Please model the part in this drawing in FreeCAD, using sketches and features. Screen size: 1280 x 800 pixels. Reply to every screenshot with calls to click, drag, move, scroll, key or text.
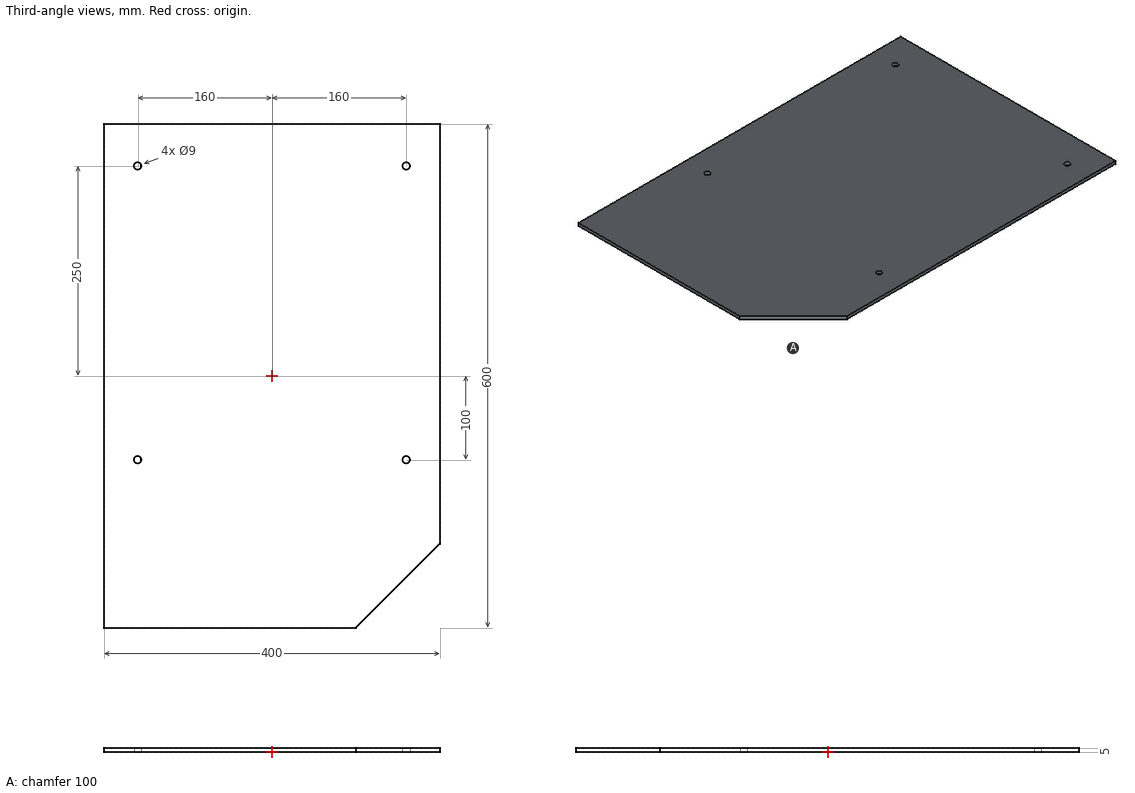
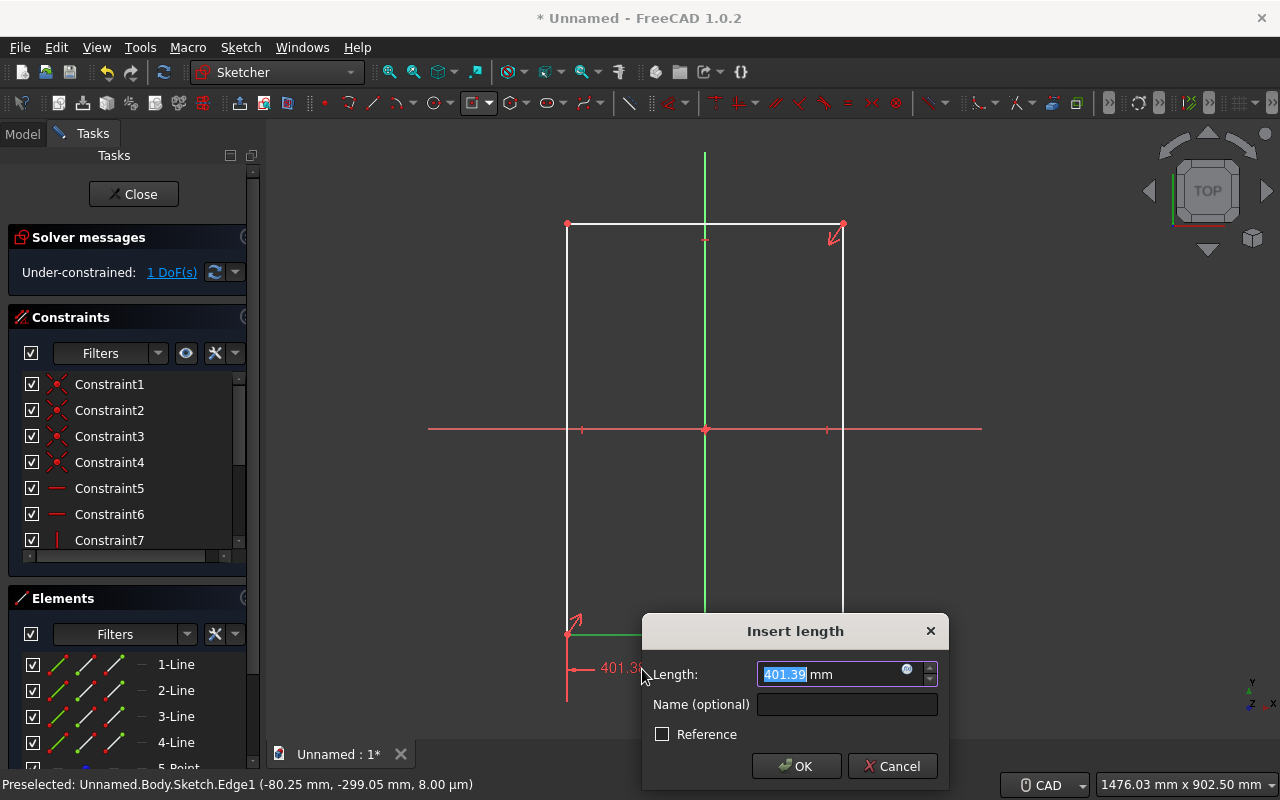
text(400)
key(Return)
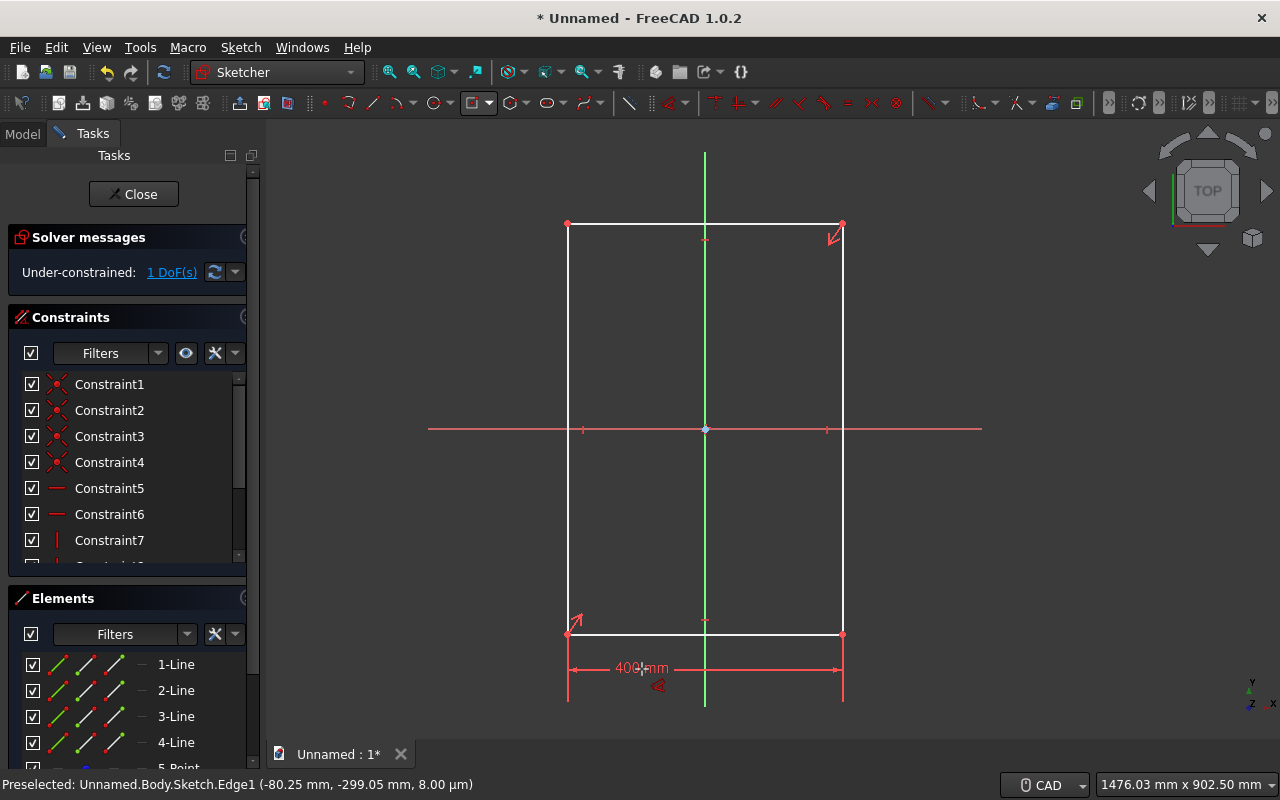
click(843, 512)
click(877, 335)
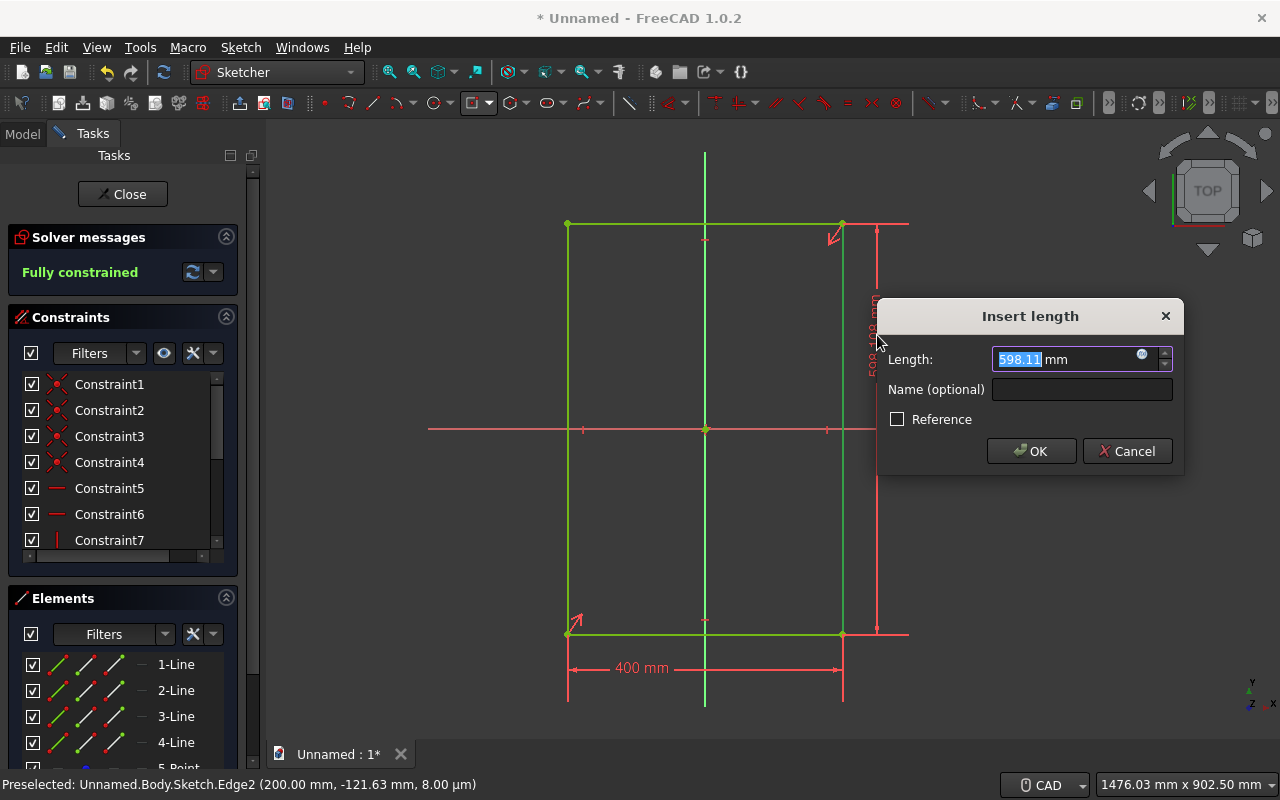
text(600)
key(Return)
key(Escape)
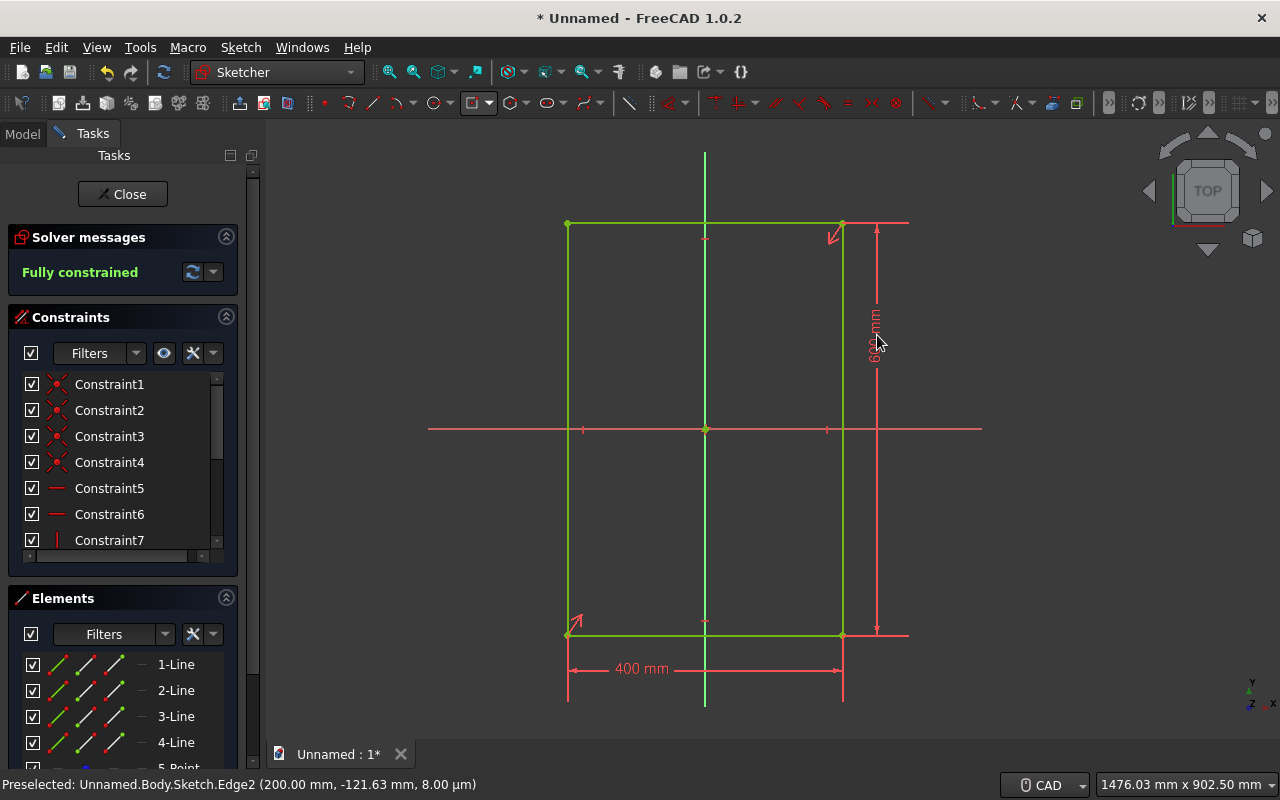
click(123, 194)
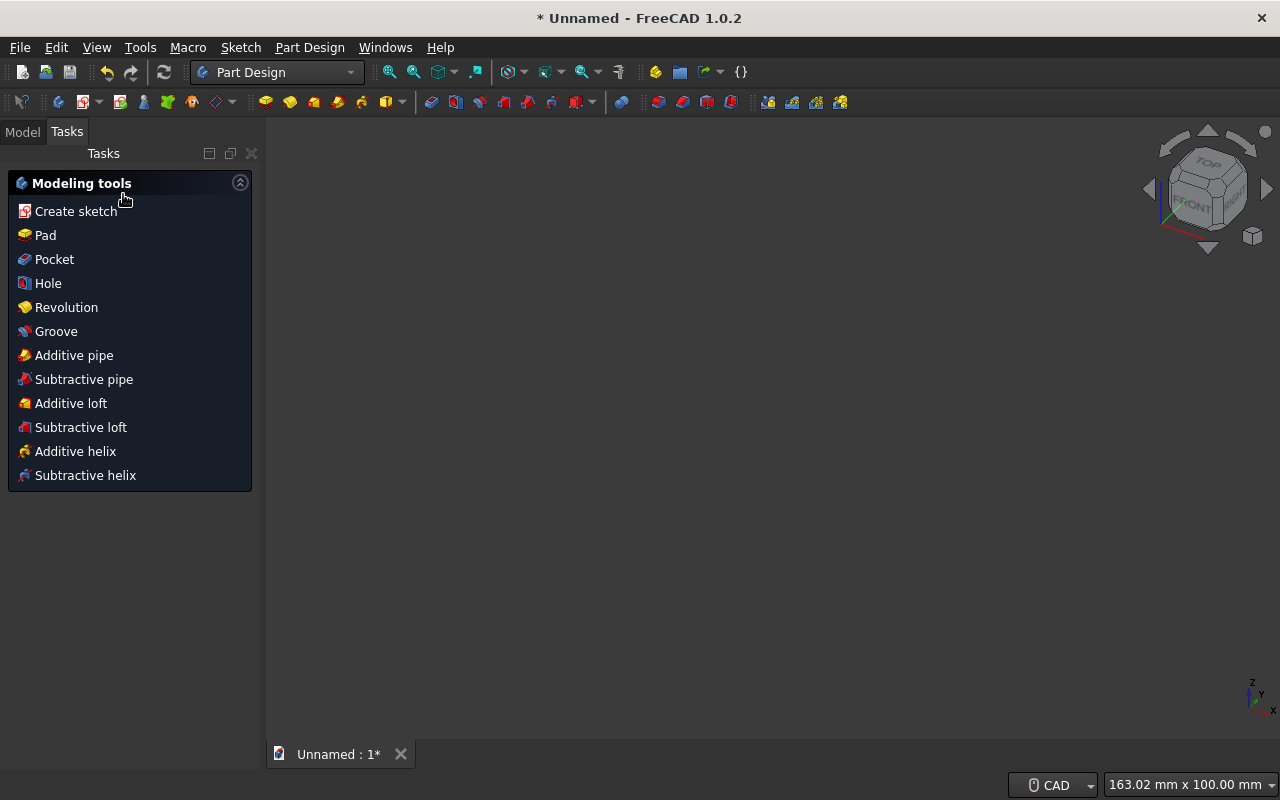
click(266, 102)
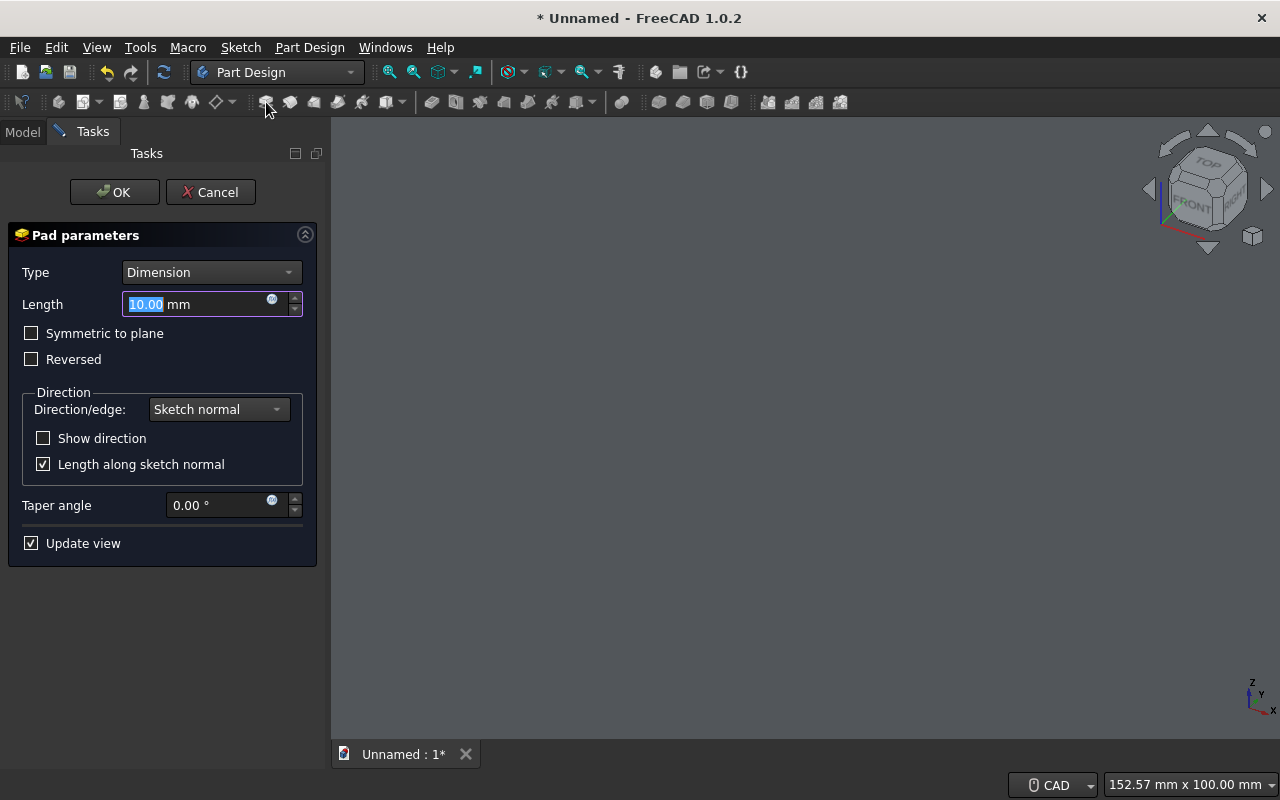
text(5)
key(Tab)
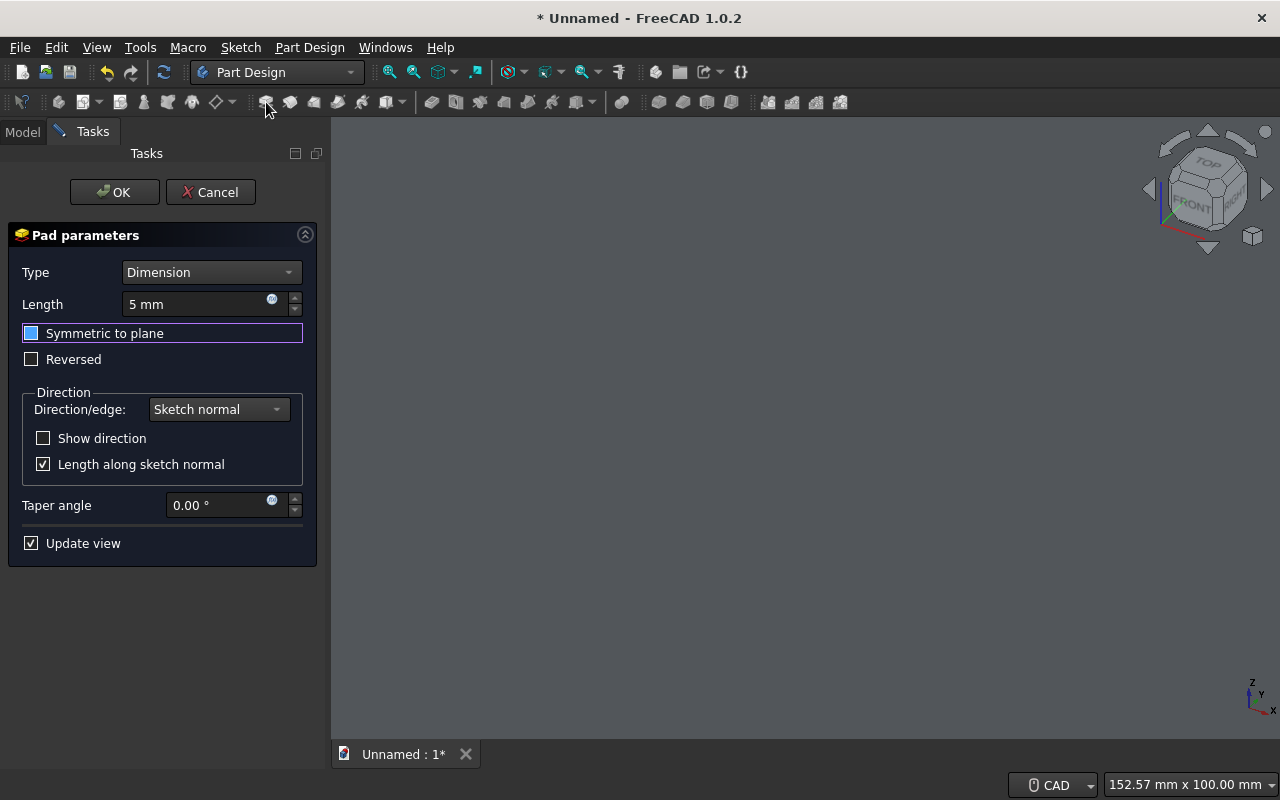
click(115, 192)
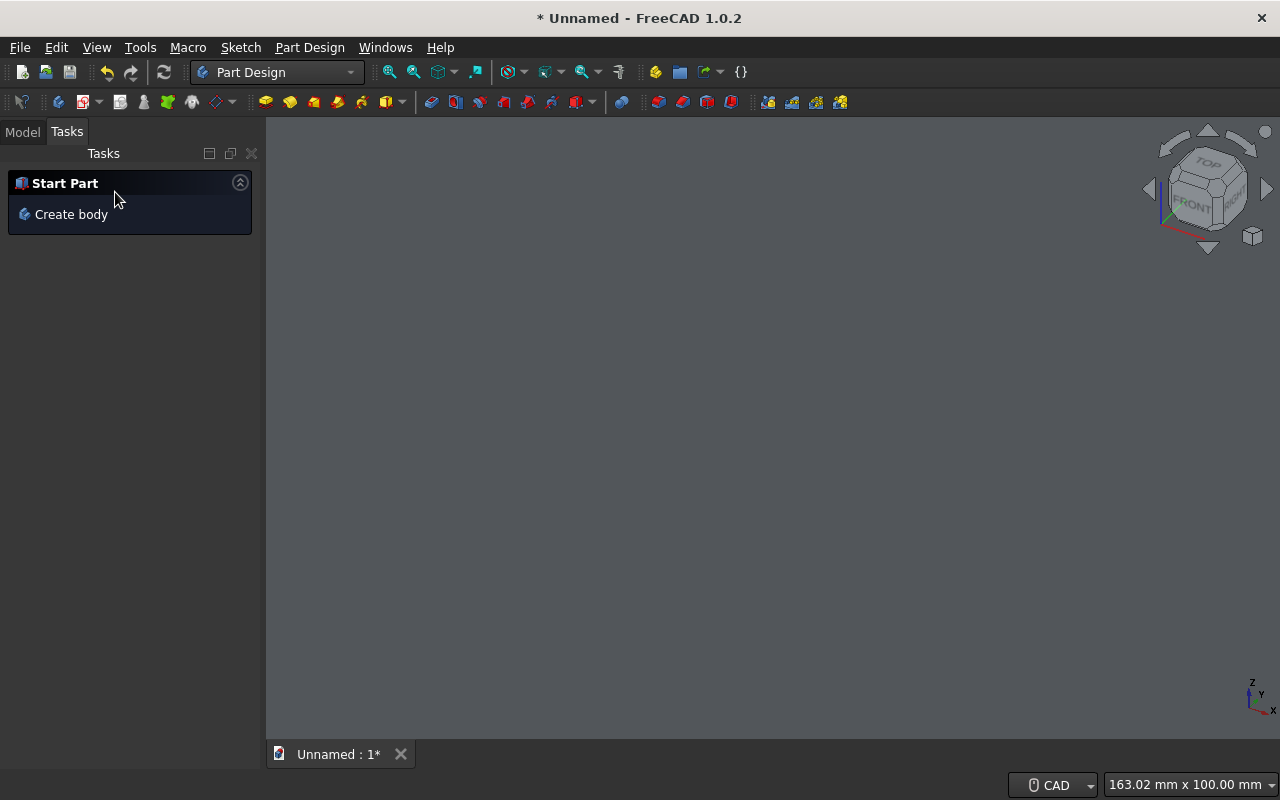
click(390, 72)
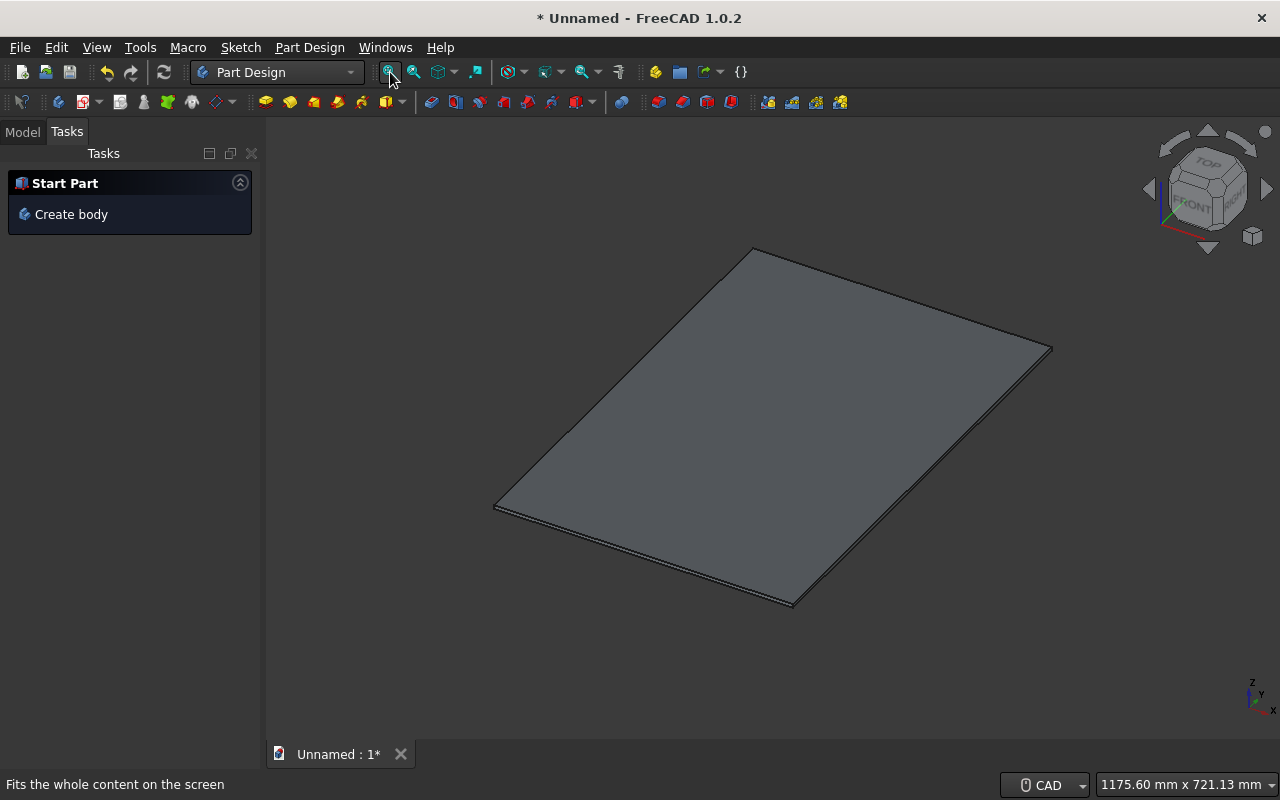
click(810, 389)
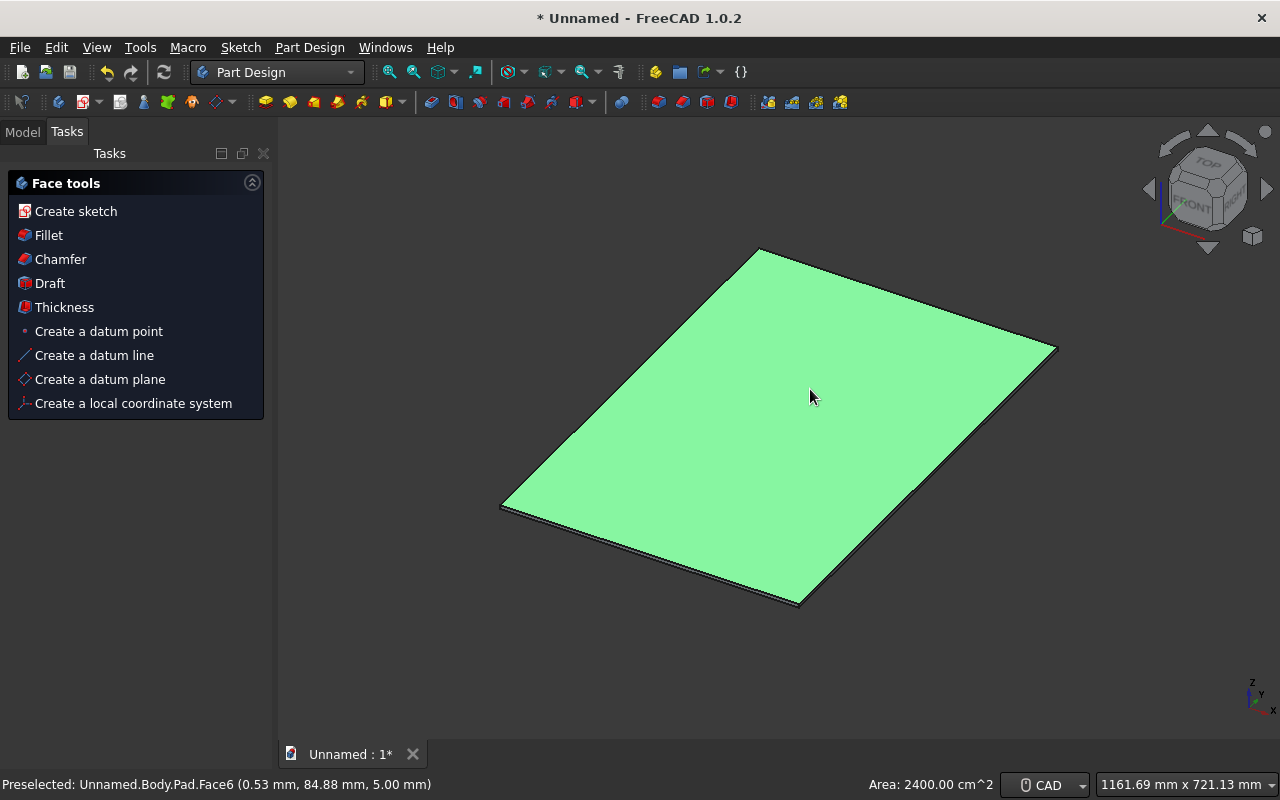
click(84, 102)